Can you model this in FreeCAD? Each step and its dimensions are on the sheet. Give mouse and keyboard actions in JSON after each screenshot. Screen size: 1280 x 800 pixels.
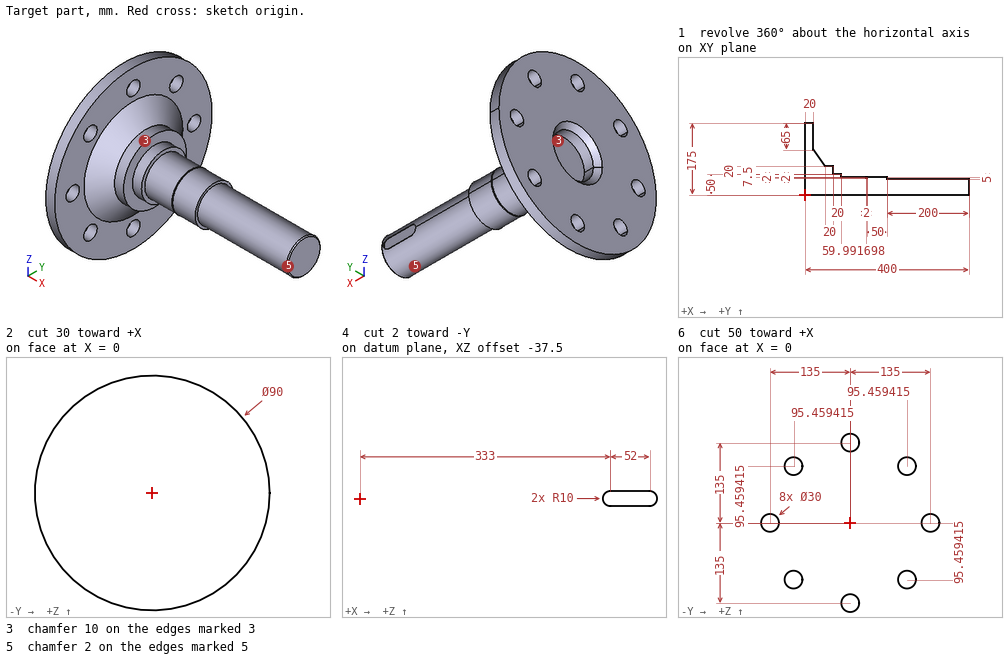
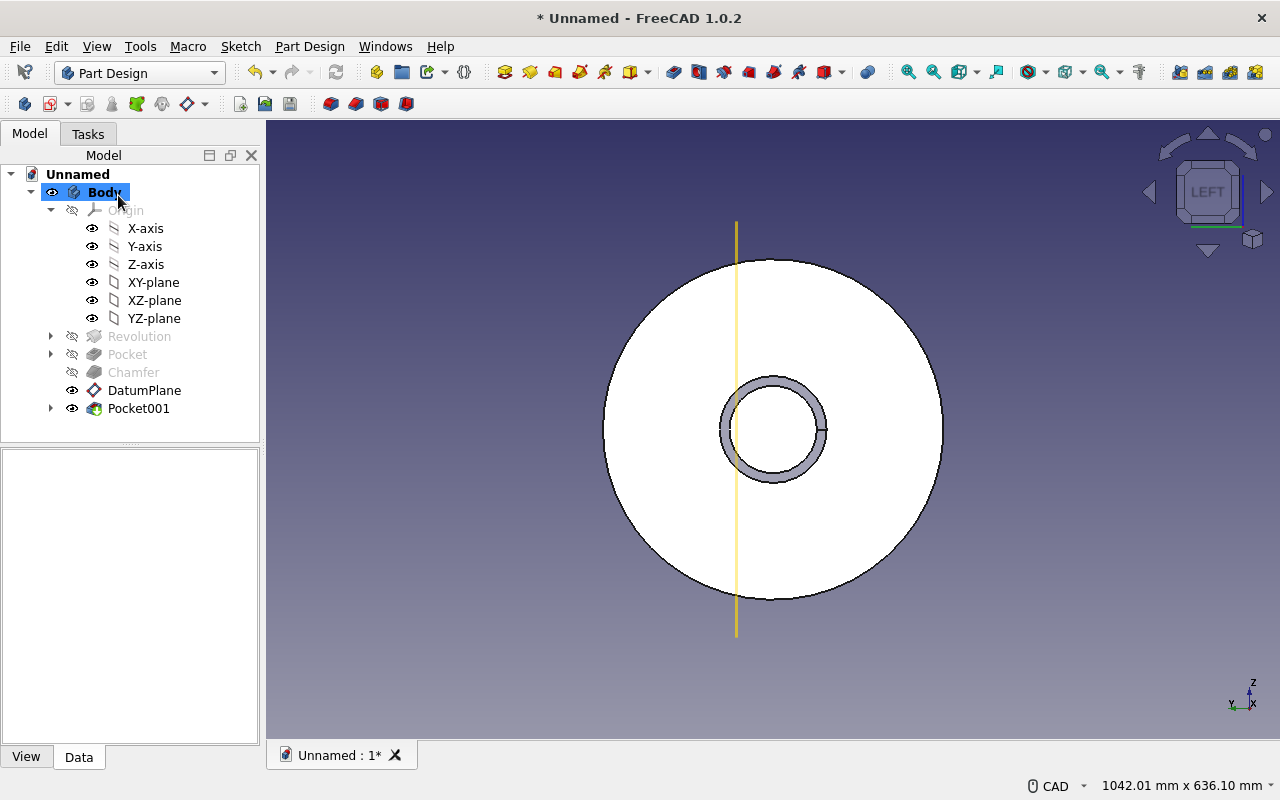
{"action": "left_click", "coordinate": [117, 390]}
{"action": "key", "text": "space"}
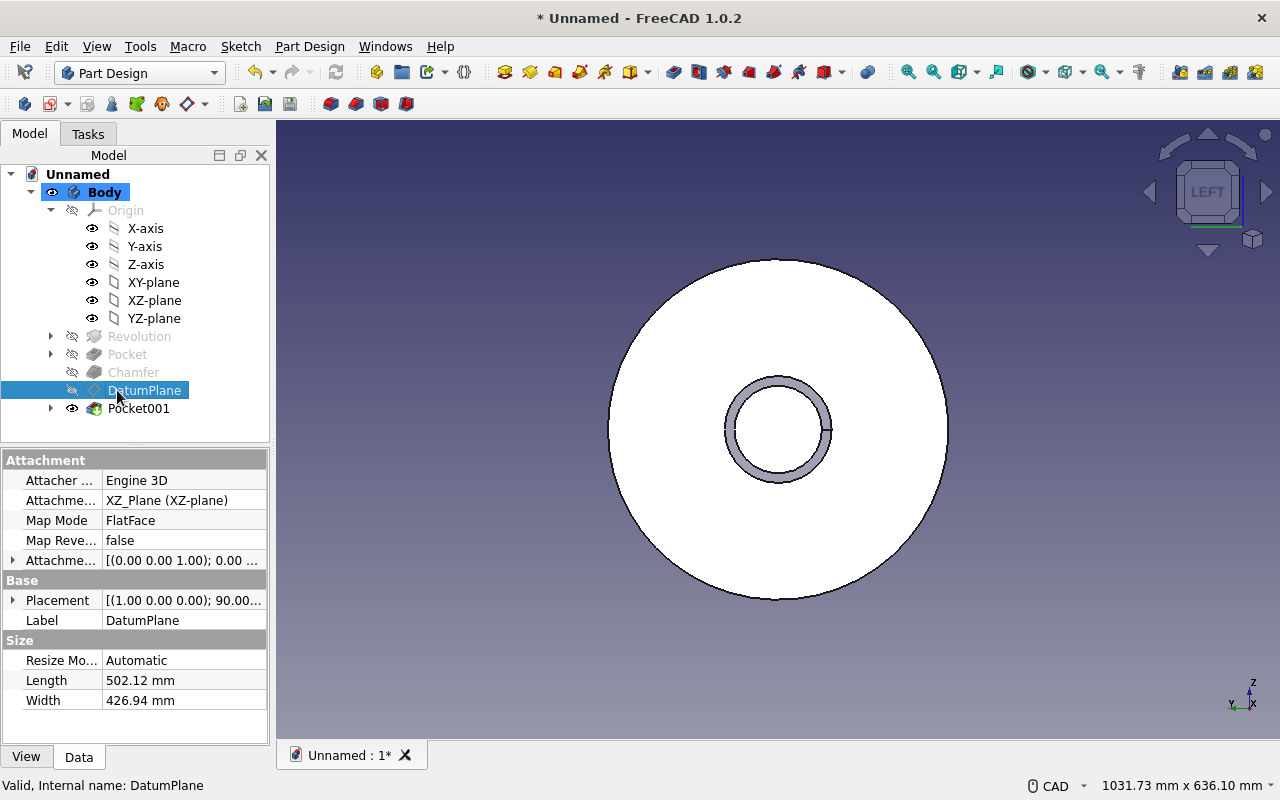
{"action": "key", "text": "0"}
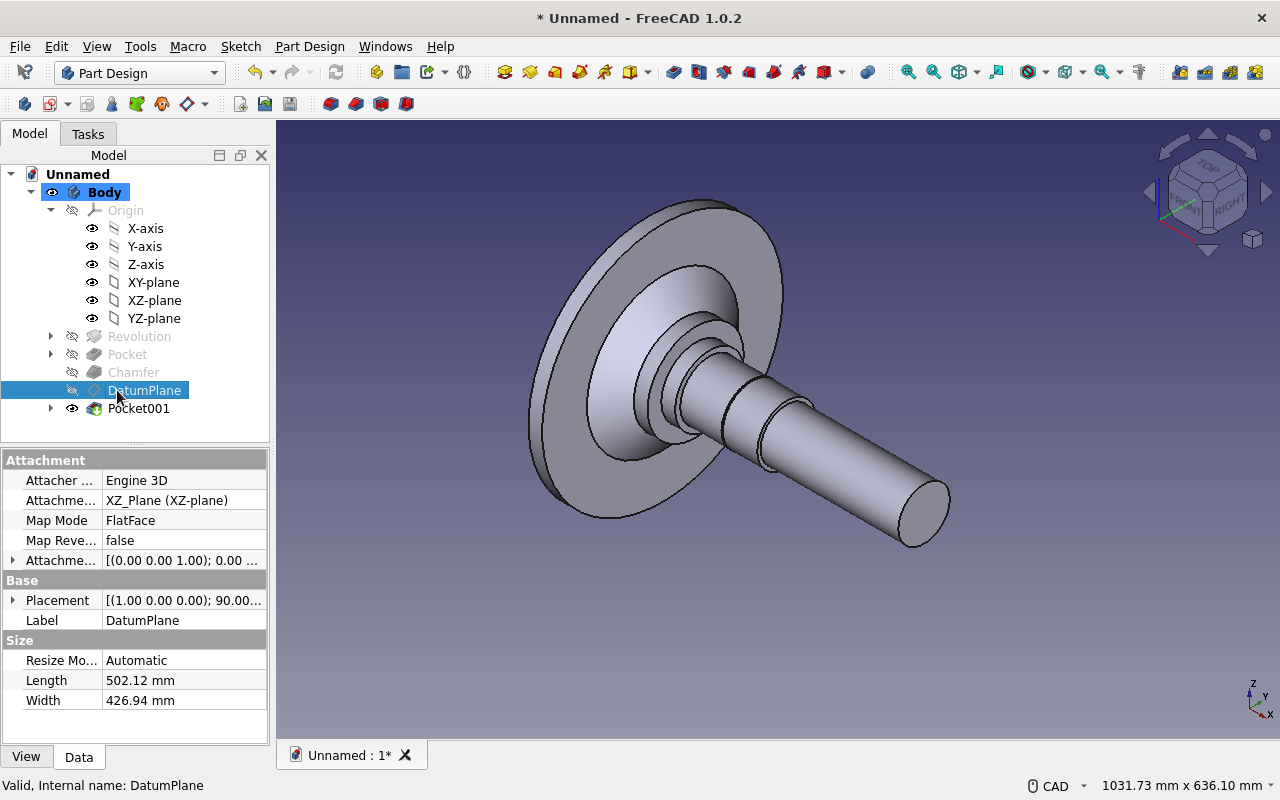
{"action": "left_click", "coordinate": [898, 528]}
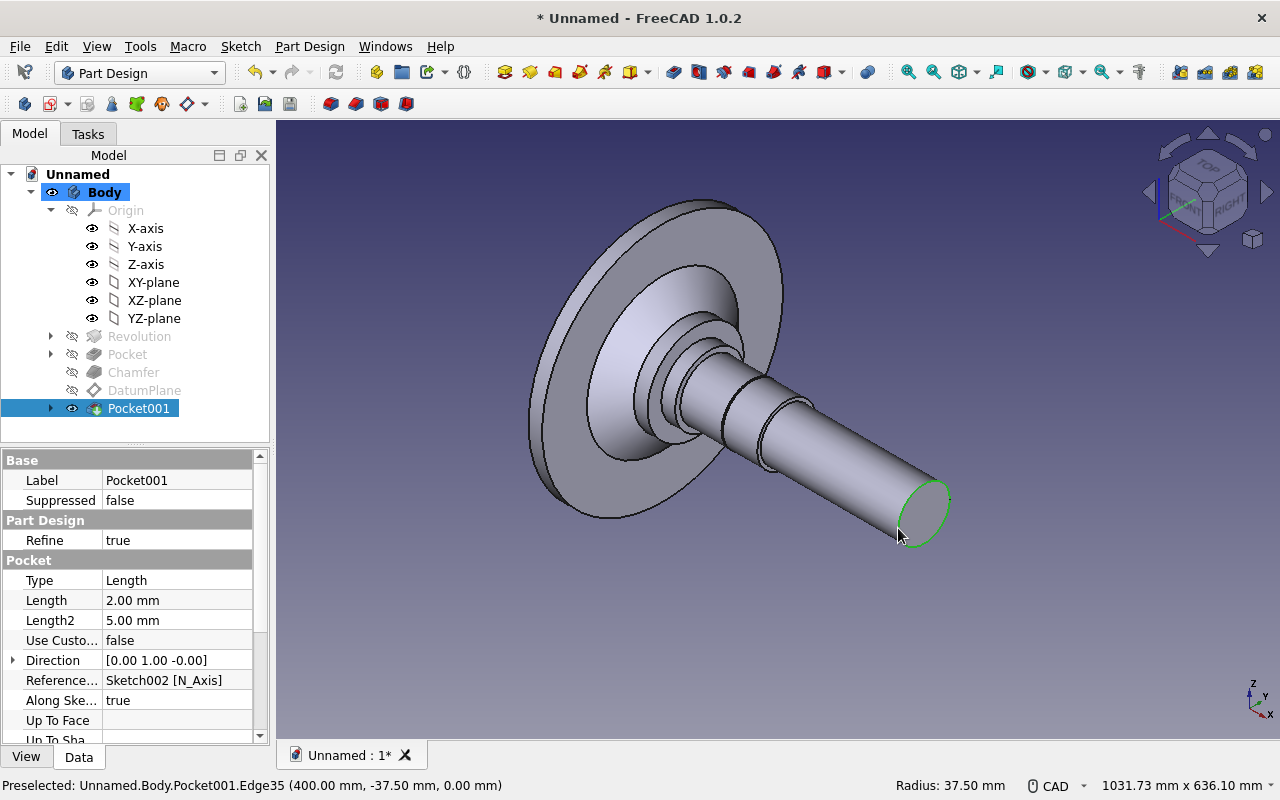
{"action": "left_click", "coordinate": [356, 104]}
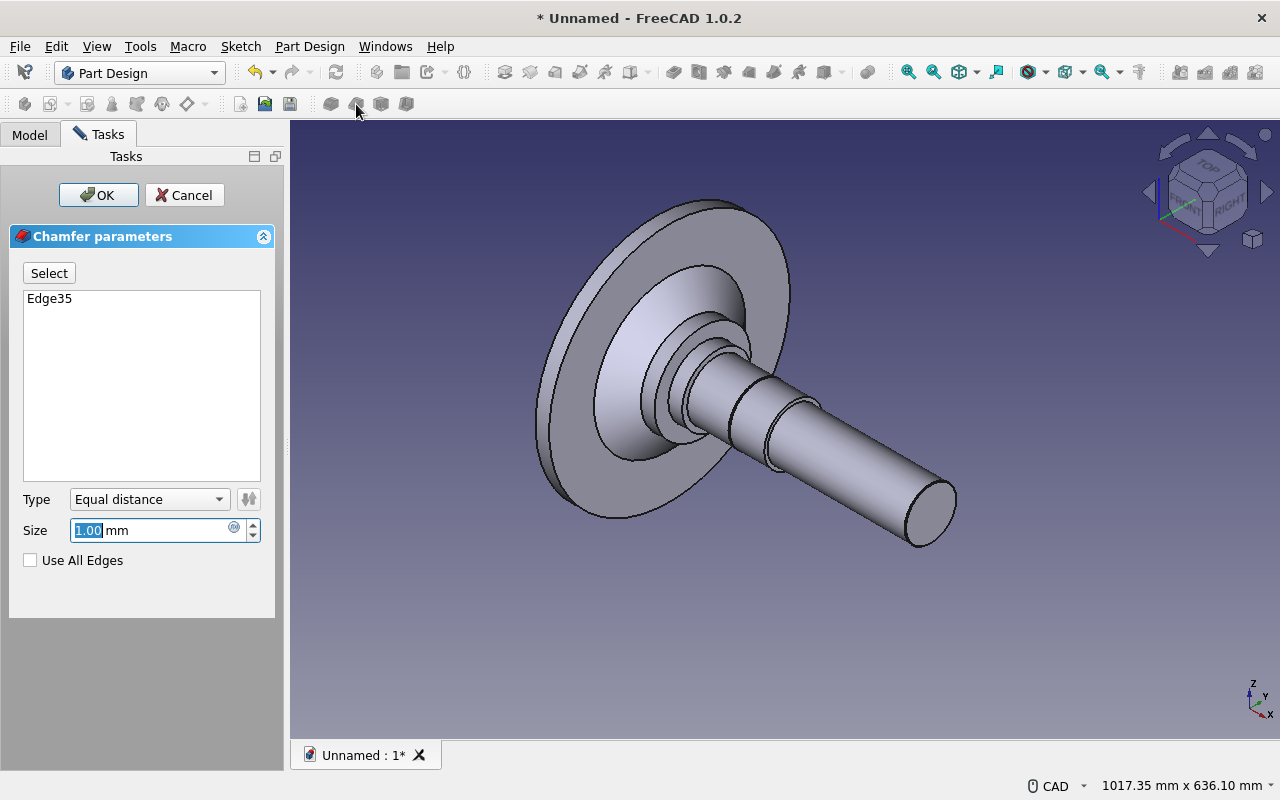
{"action": "type", "text": "2"}
{"action": "key", "text": "Tab"}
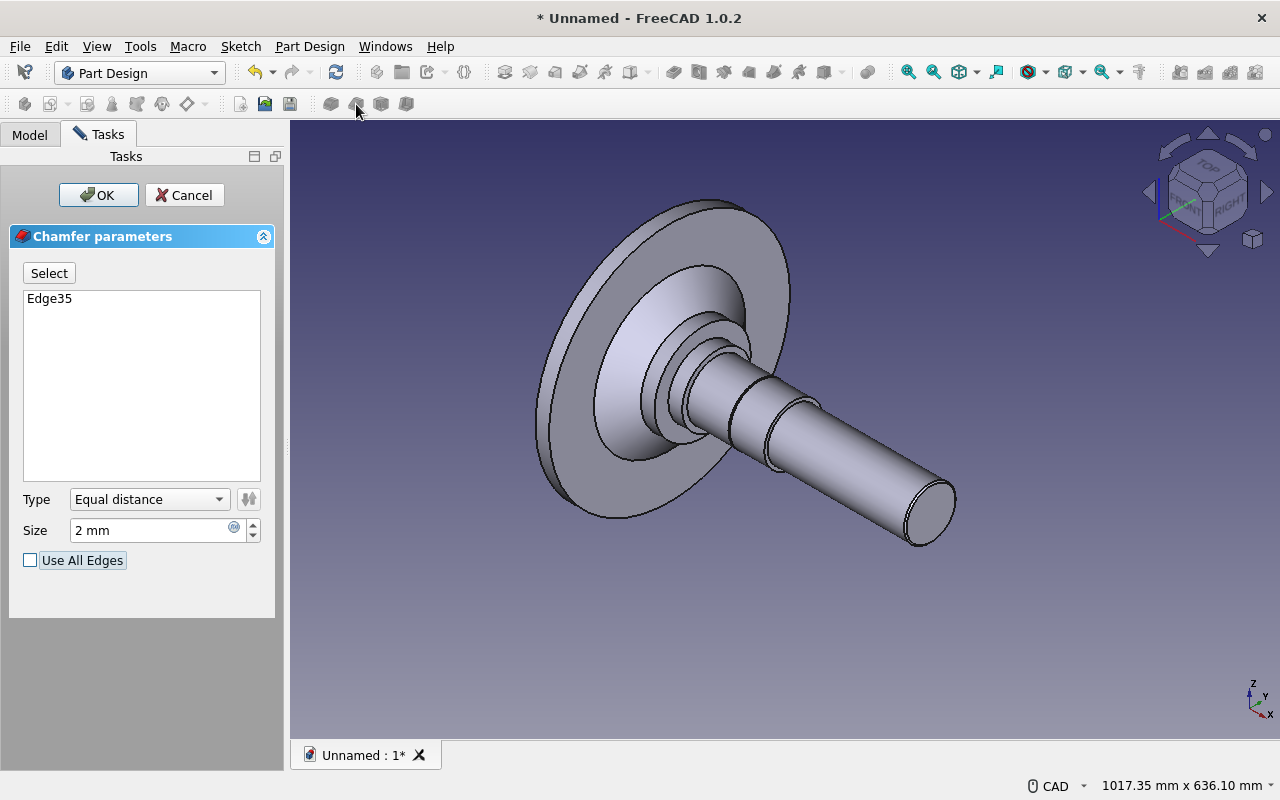
{"action": "left_click", "coordinate": [99, 195]}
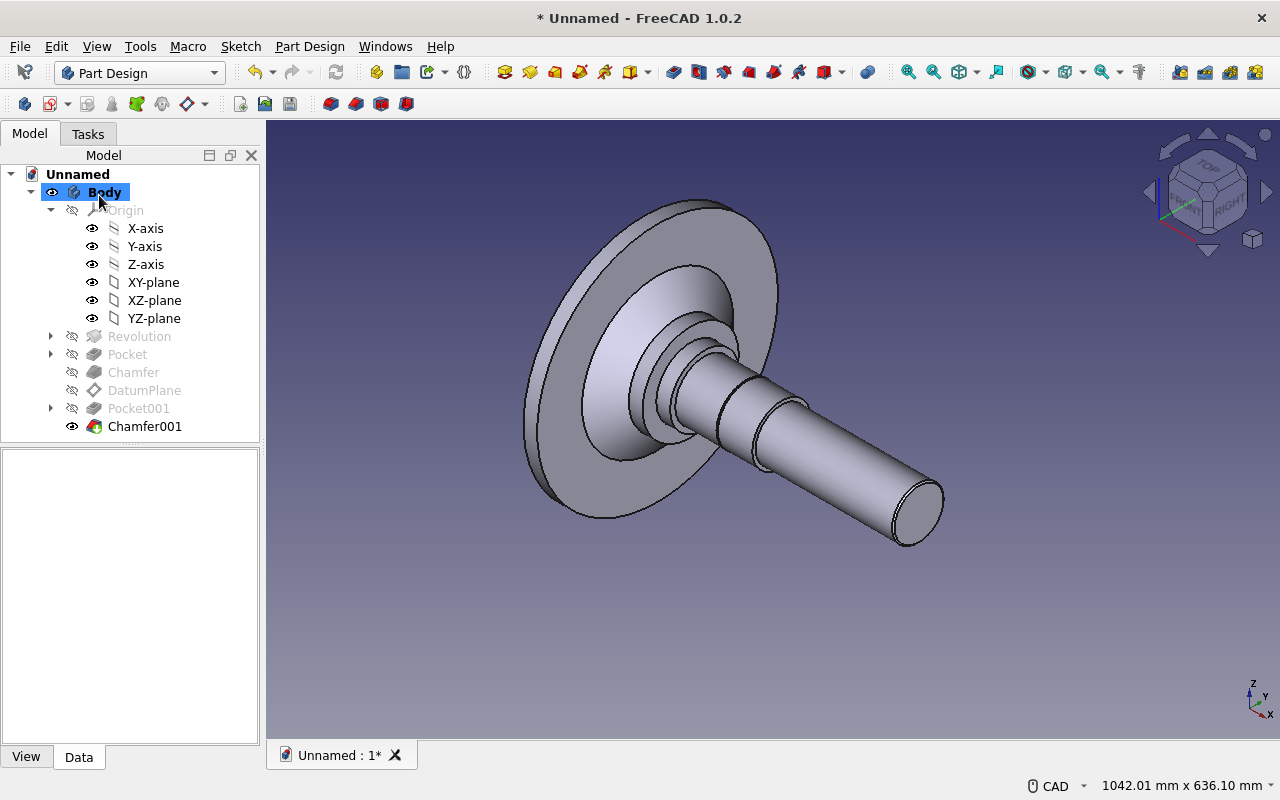
{"action": "key", "text": "6"}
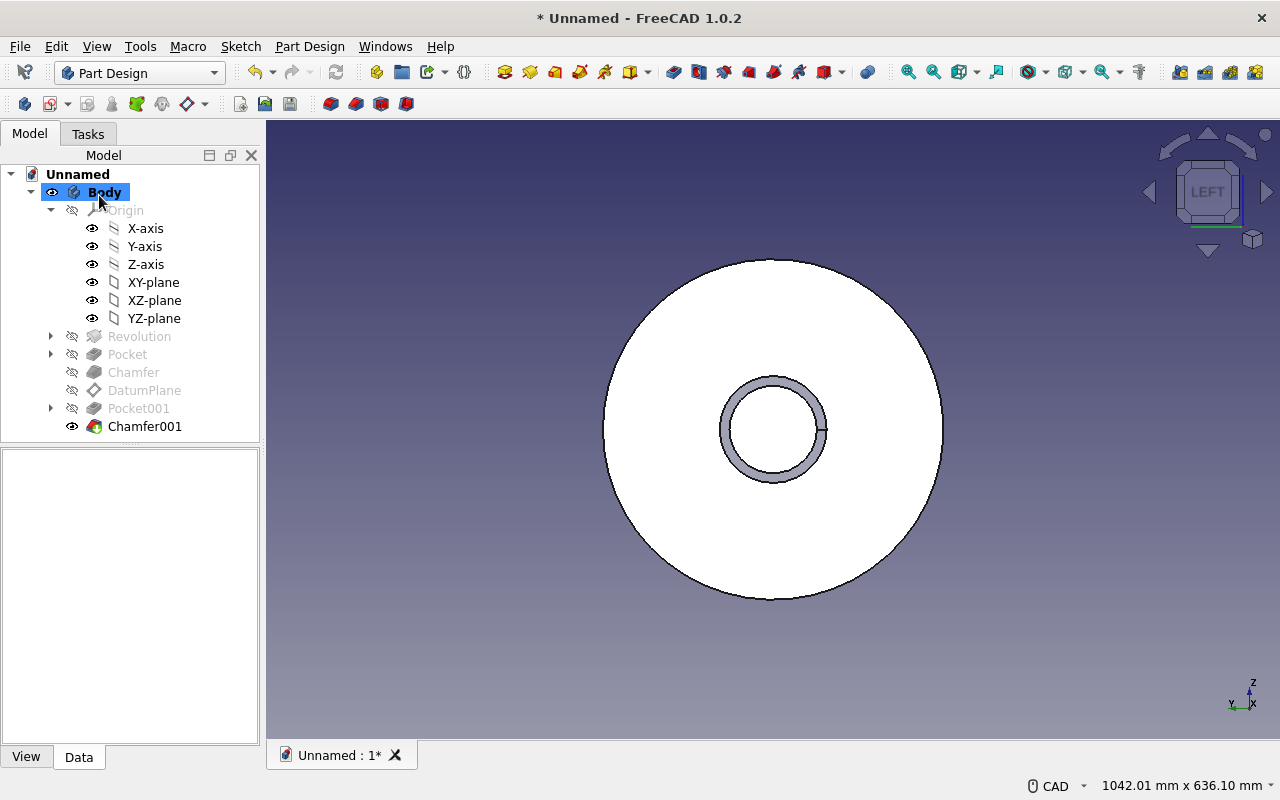
{"action": "left_click", "coordinate": [725, 331]}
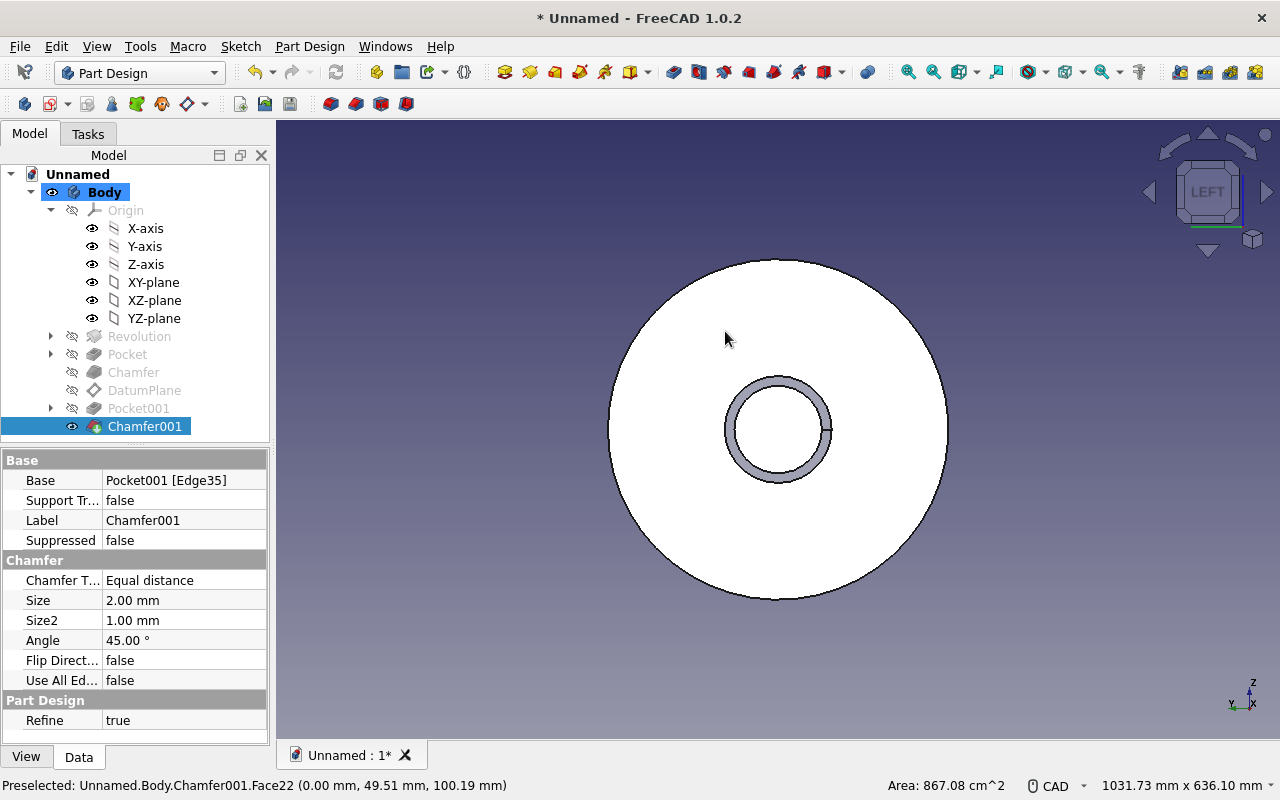
{"action": "left_click", "coordinate": [50, 104]}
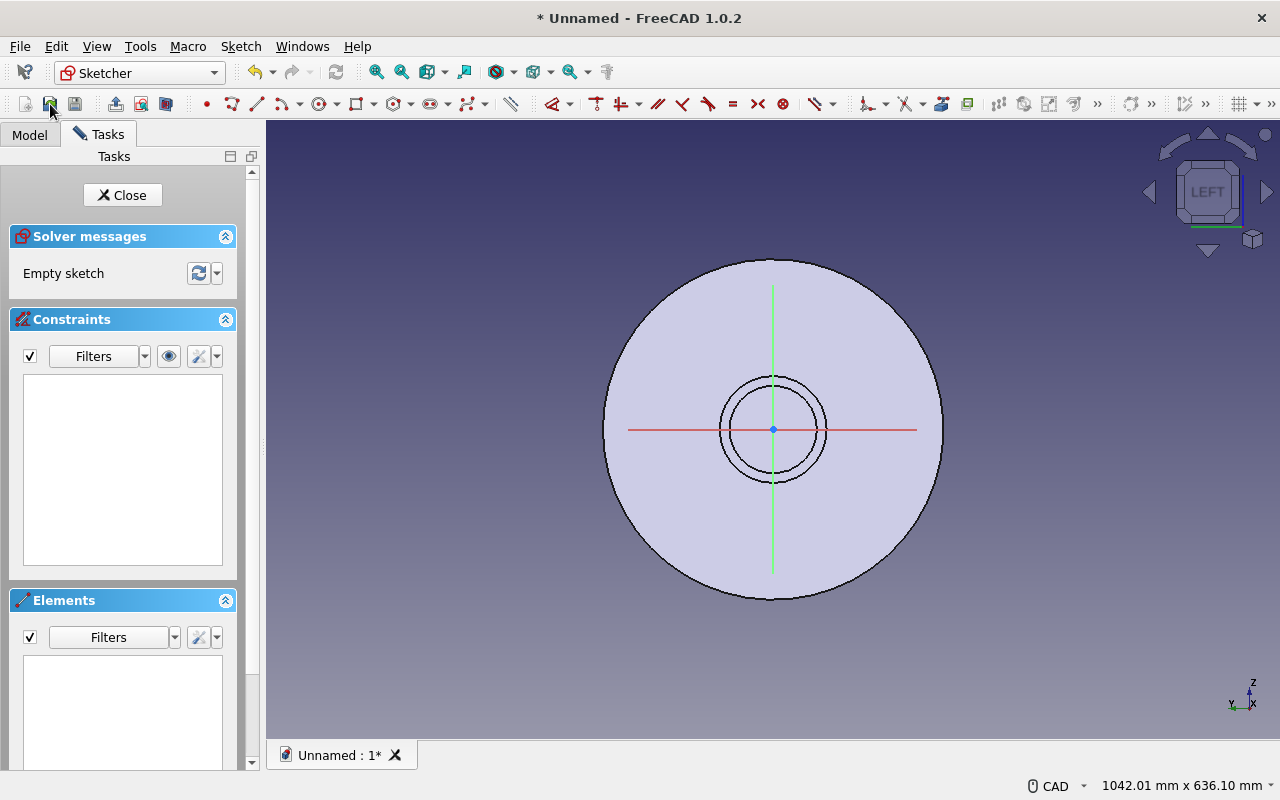
{"action": "scroll", "coordinate": [913, 430], "scroll_direction": "up", "scroll_amount": 2}